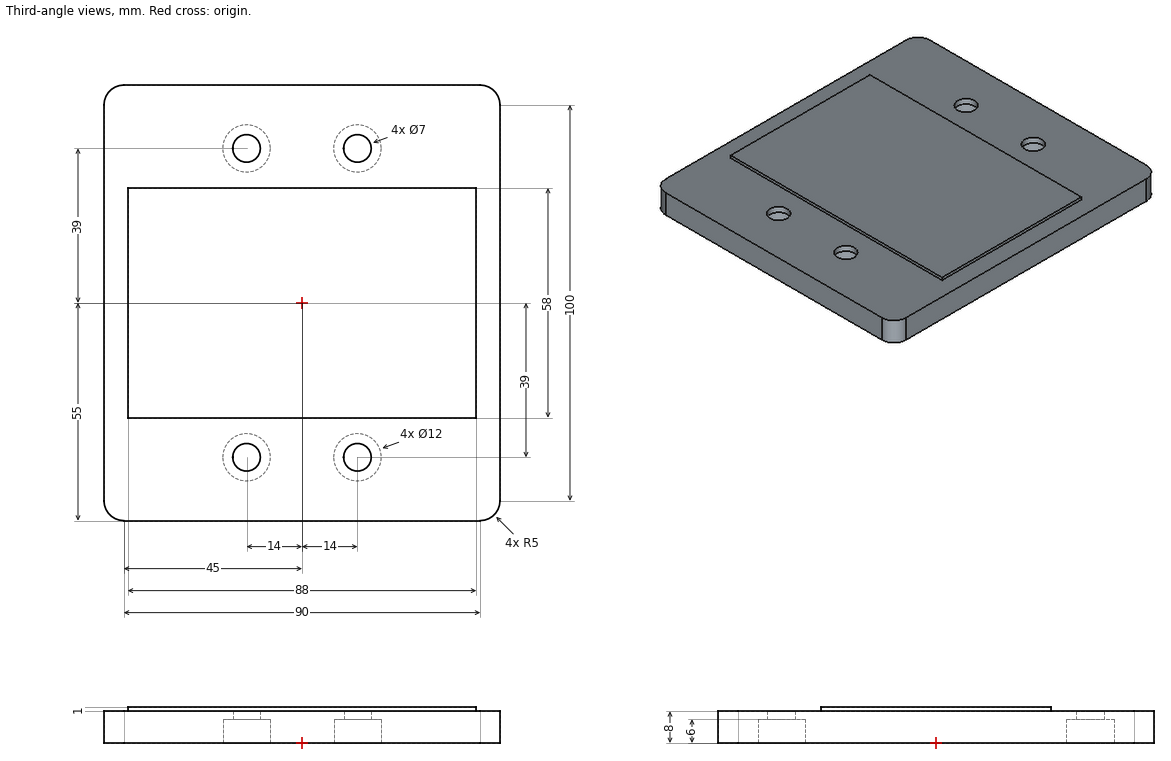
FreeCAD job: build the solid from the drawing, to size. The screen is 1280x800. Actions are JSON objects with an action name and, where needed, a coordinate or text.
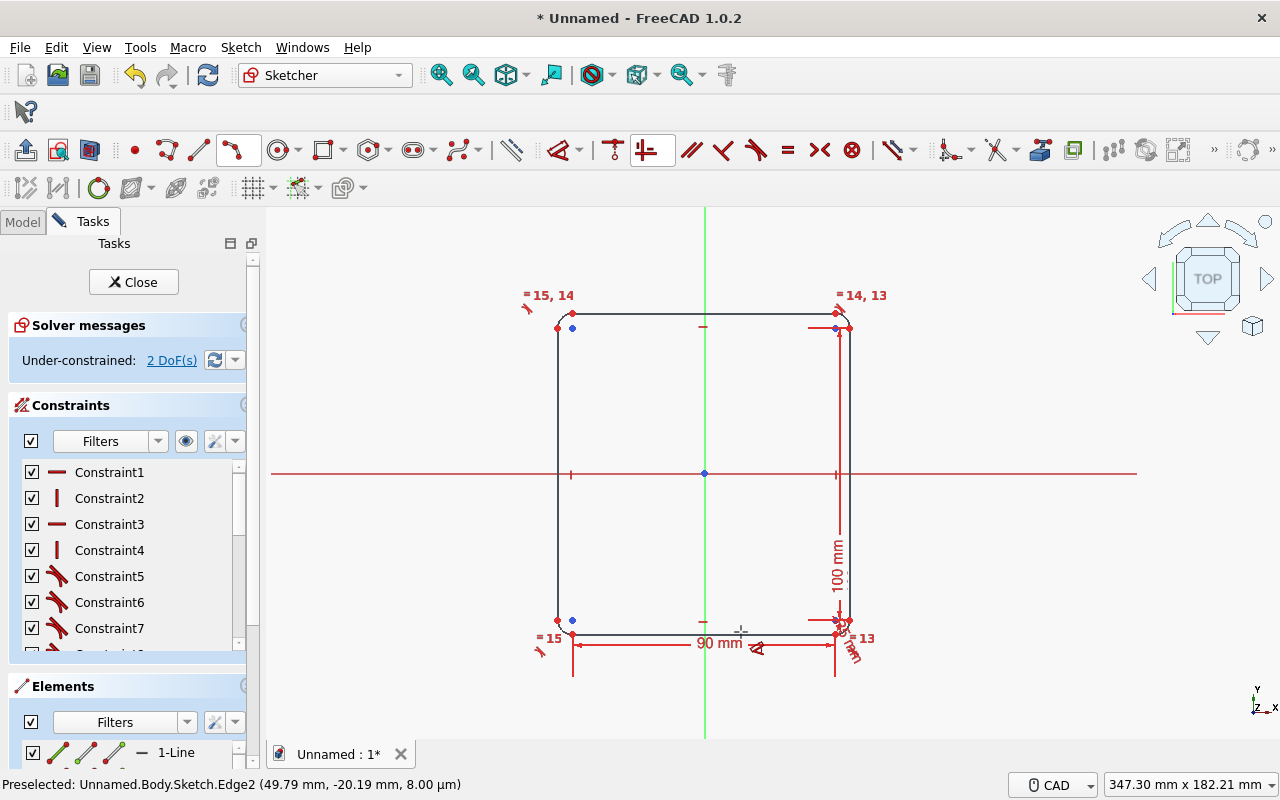
{"action": "left_click", "coordinate": [573, 635]}
{"action": "left_click", "coordinate": [639, 669]}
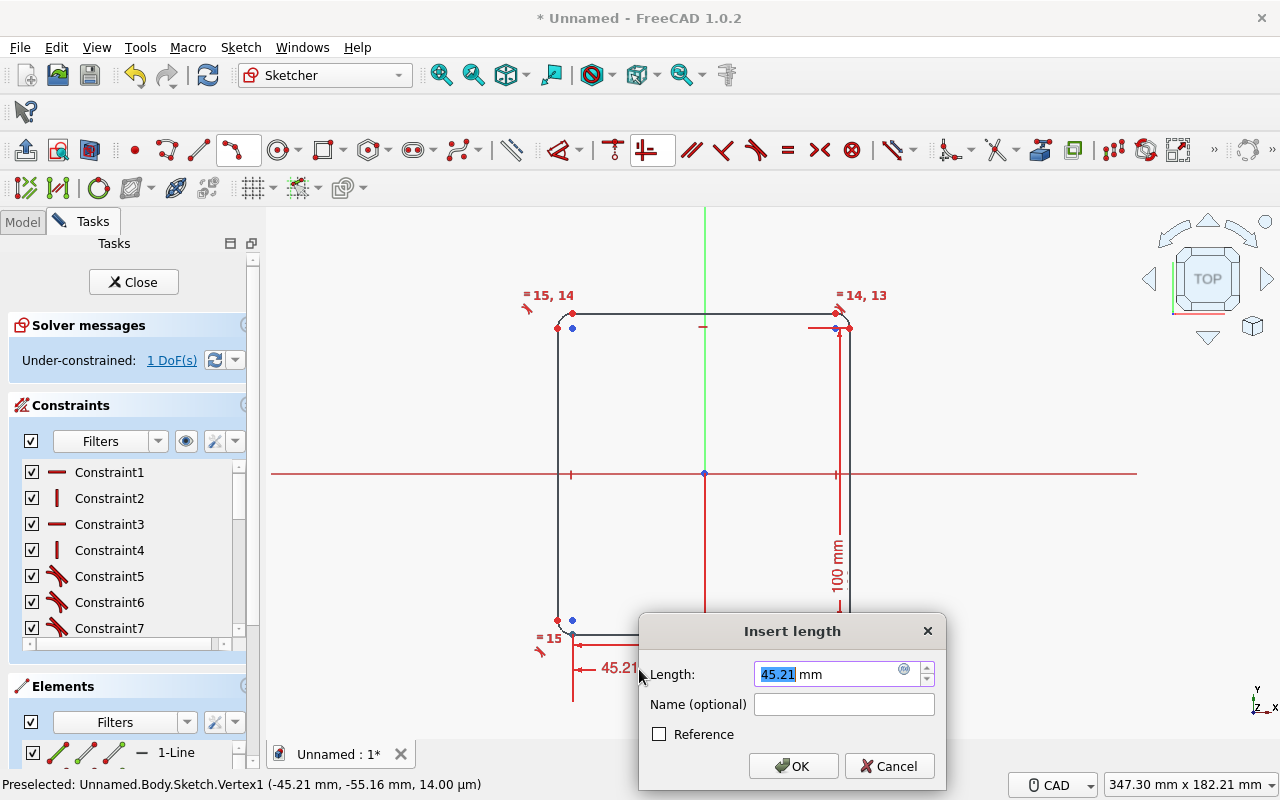
{"action": "type", "text": "45"}
{"action": "key", "text": "Return"}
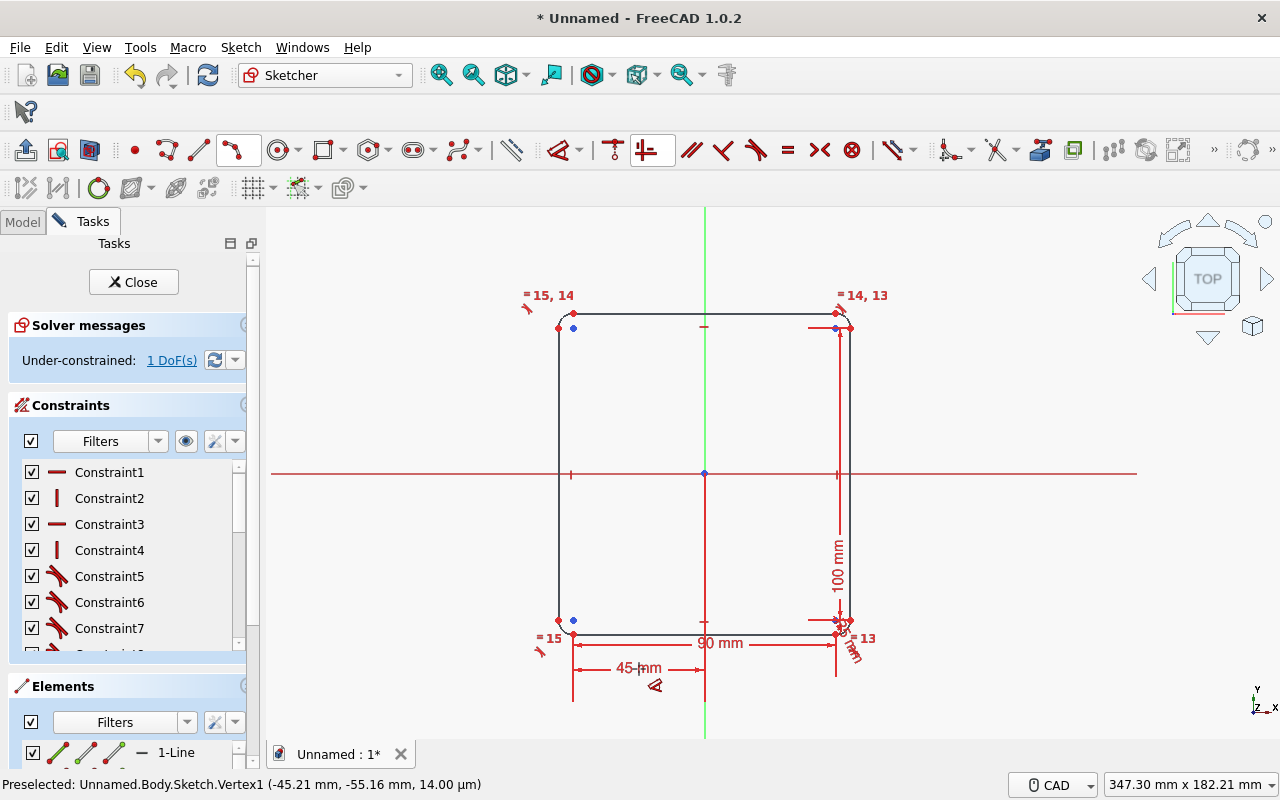
{"action": "left_click", "coordinate": [573, 635]}
{"action": "left_click", "coordinate": [539, 554]}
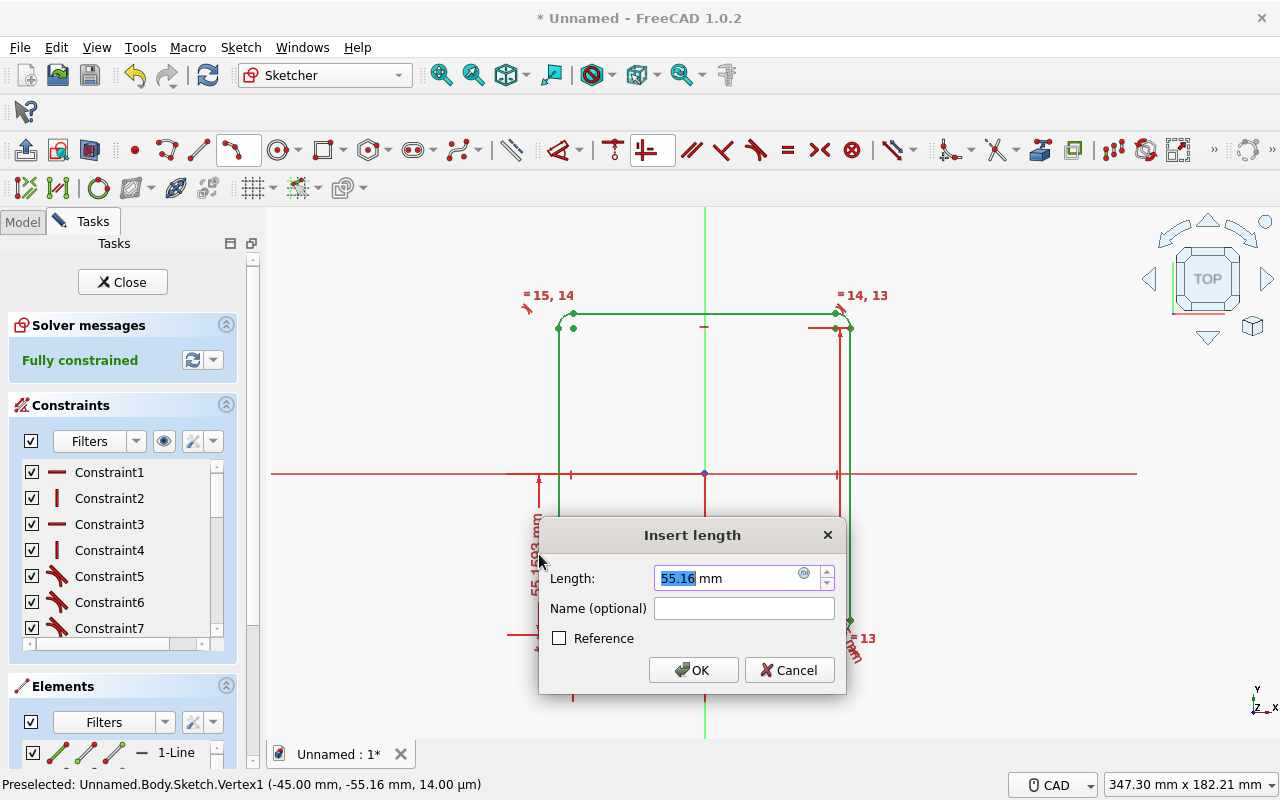
{"action": "type", "text": "55"}
{"action": "key", "text": "Return"}
{"action": "key", "text": "Escape"}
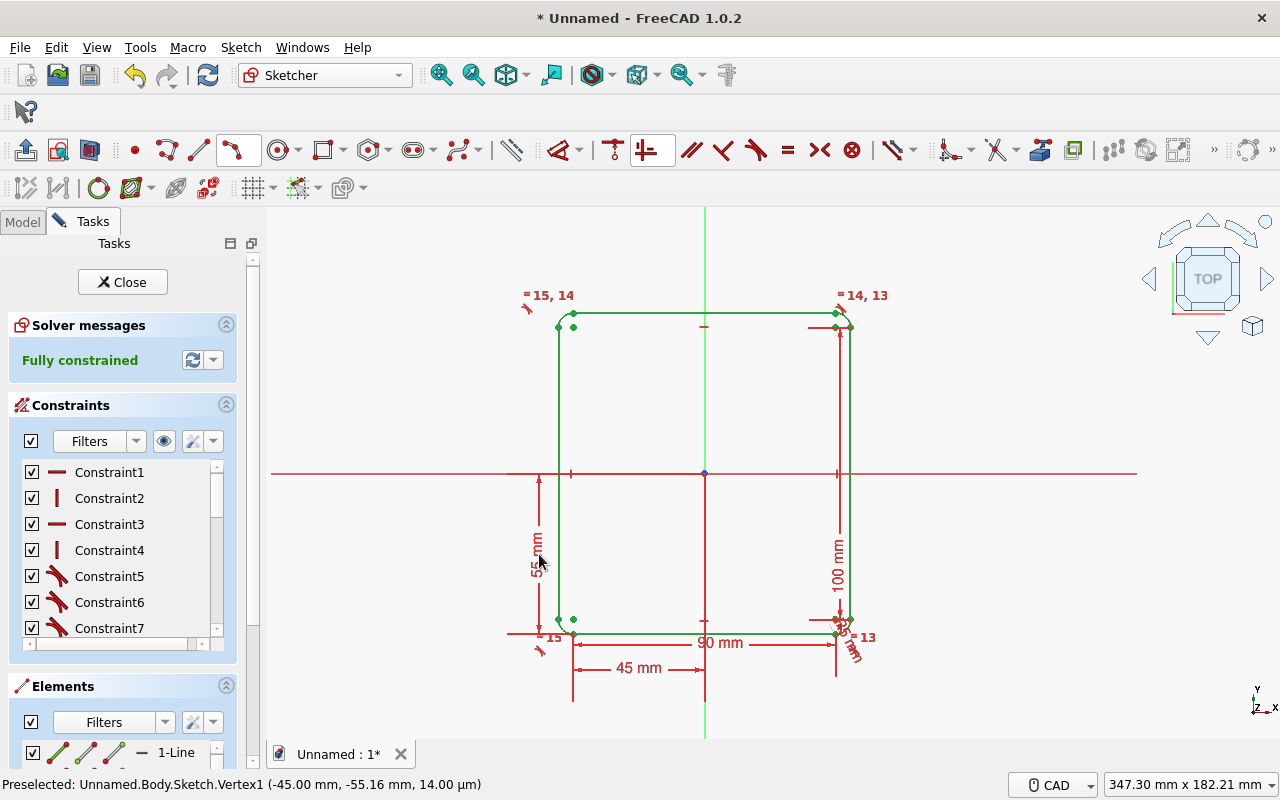
{"action": "left_click", "coordinate": [123, 282]}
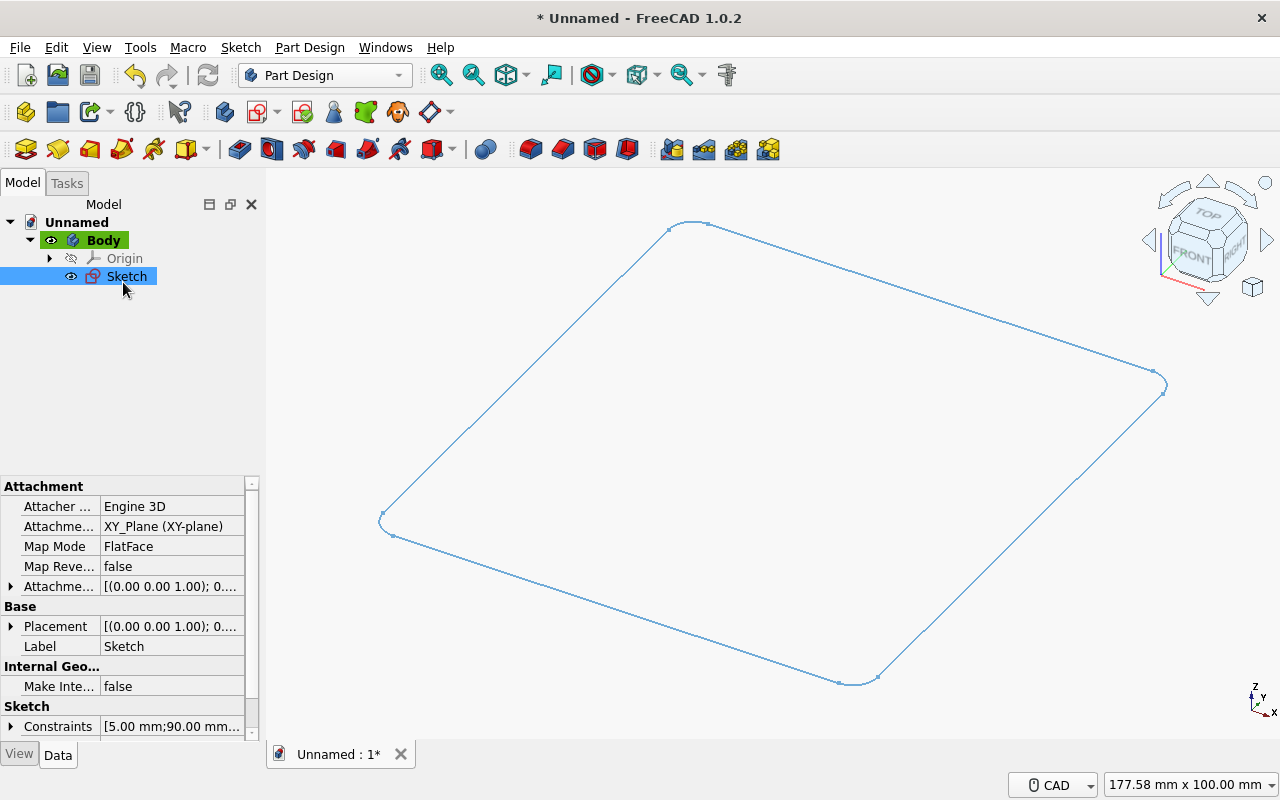
{"action": "left_click", "coordinate": [26, 150]}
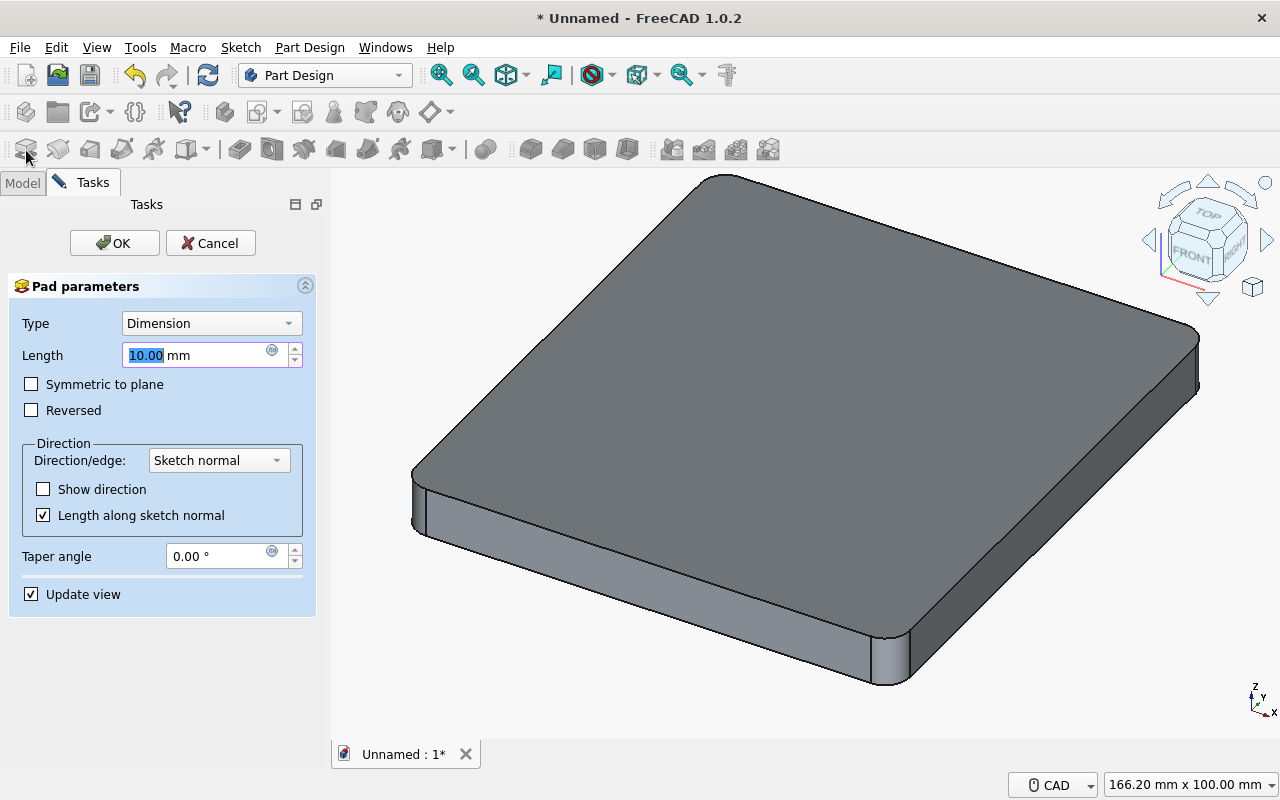
{"action": "type", "text": "8"}
{"action": "key", "text": "Tab"}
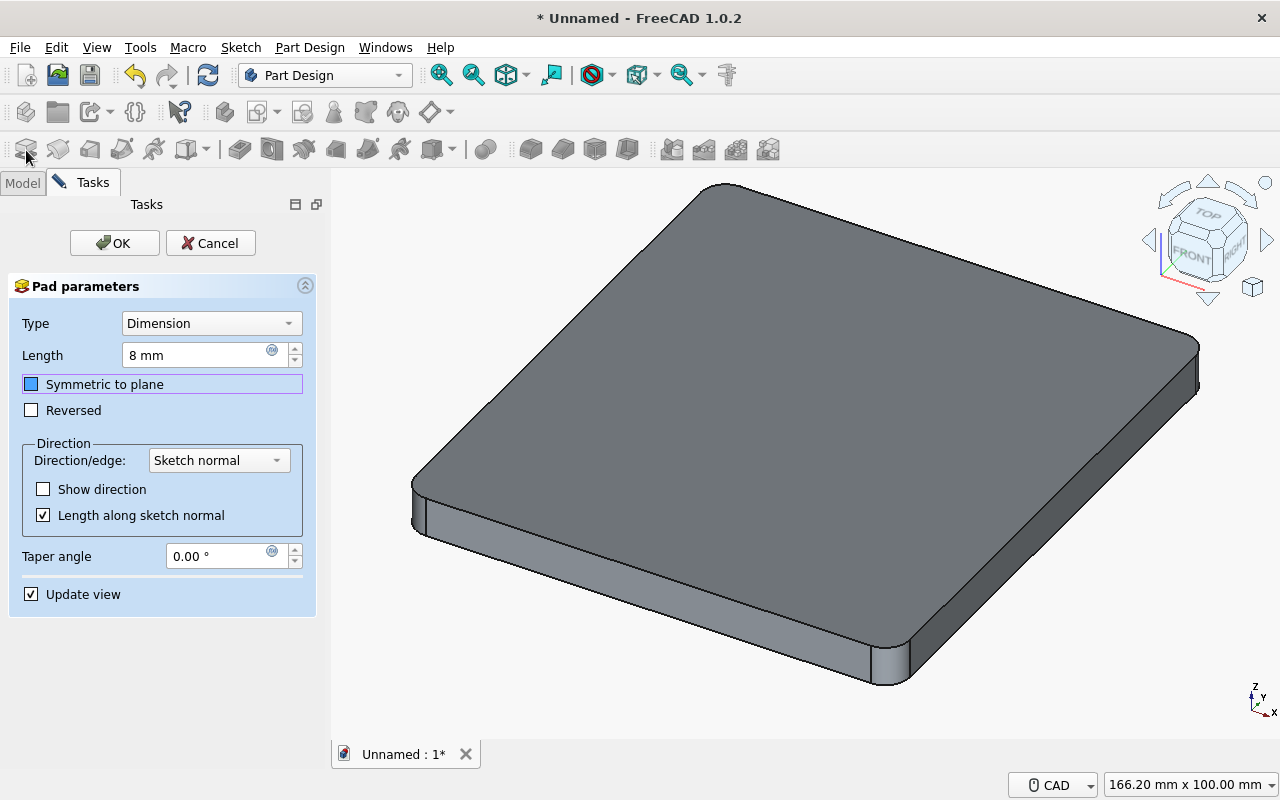
{"action": "left_click", "coordinate": [115, 243]}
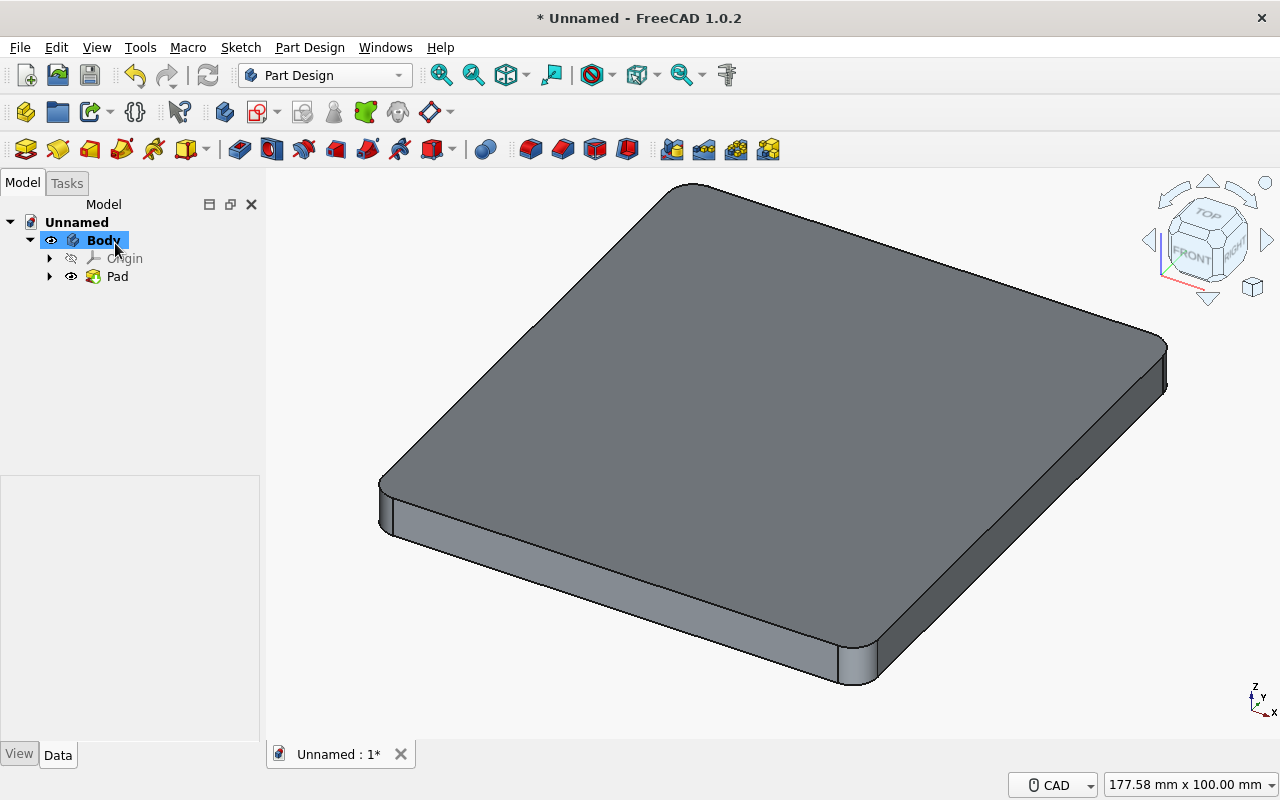
{"action": "left_click", "coordinate": [773, 415]}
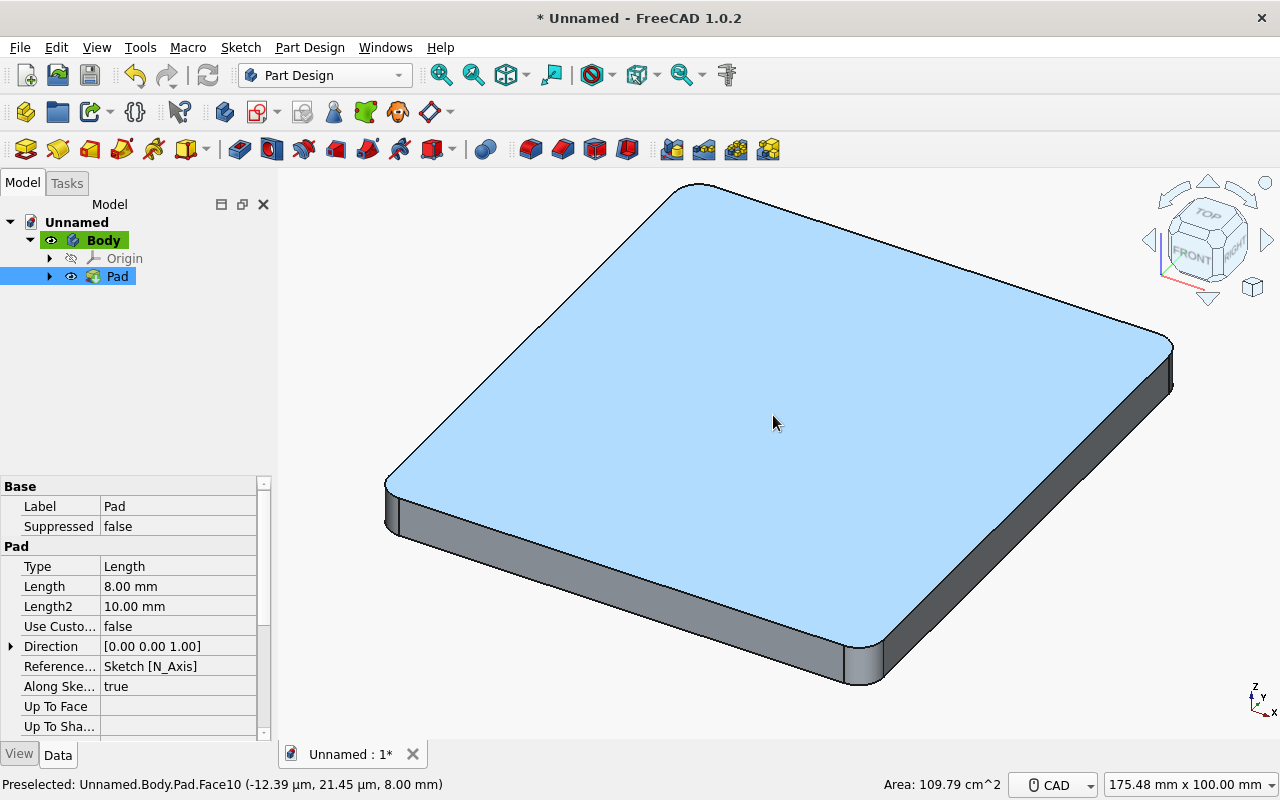
{"action": "left_click", "coordinate": [258, 112]}